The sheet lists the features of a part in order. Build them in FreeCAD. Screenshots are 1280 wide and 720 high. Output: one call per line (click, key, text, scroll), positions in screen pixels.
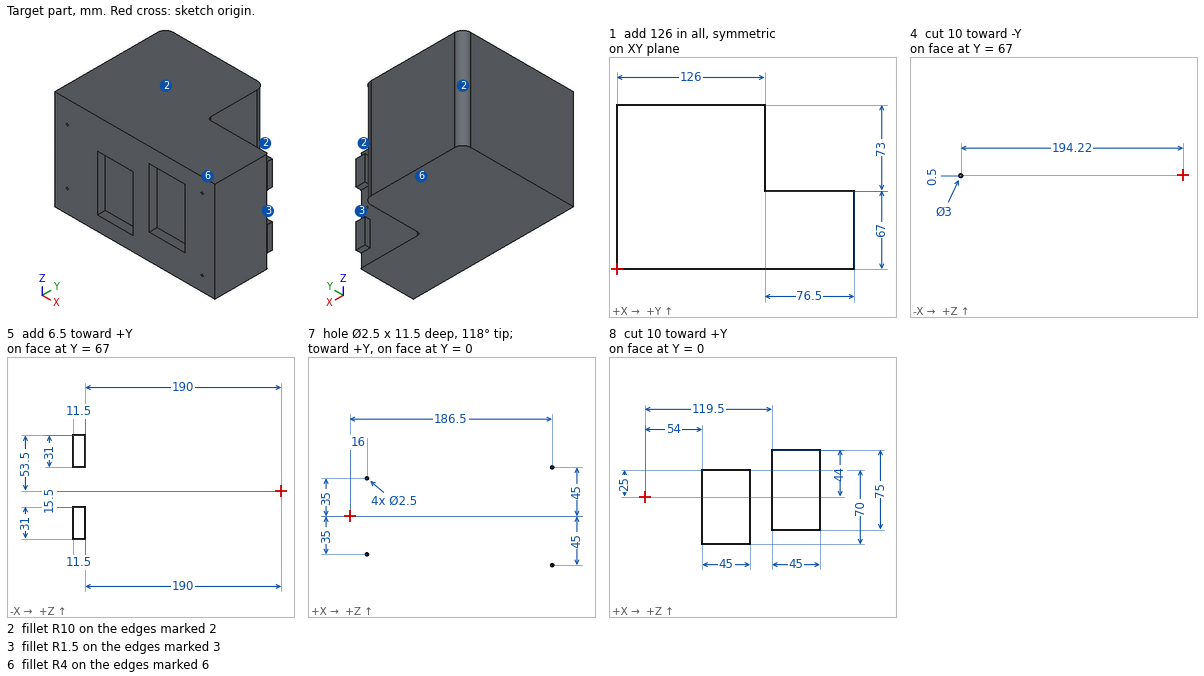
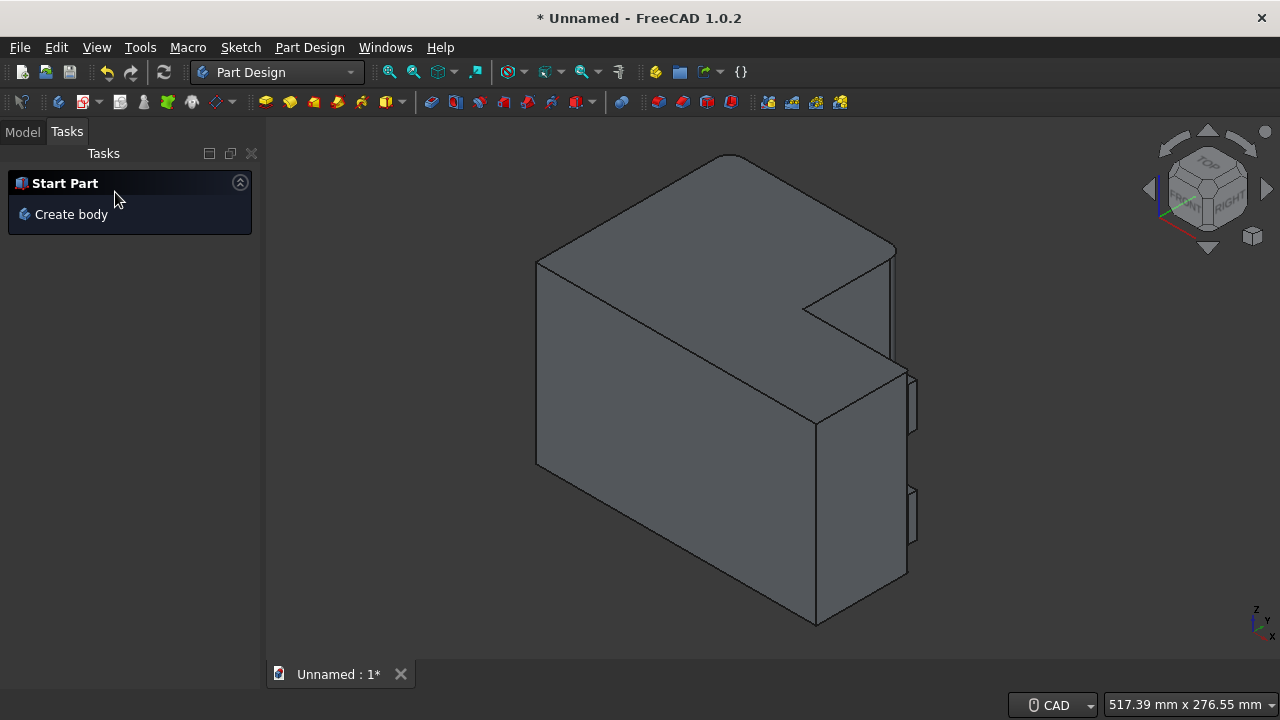
key(2)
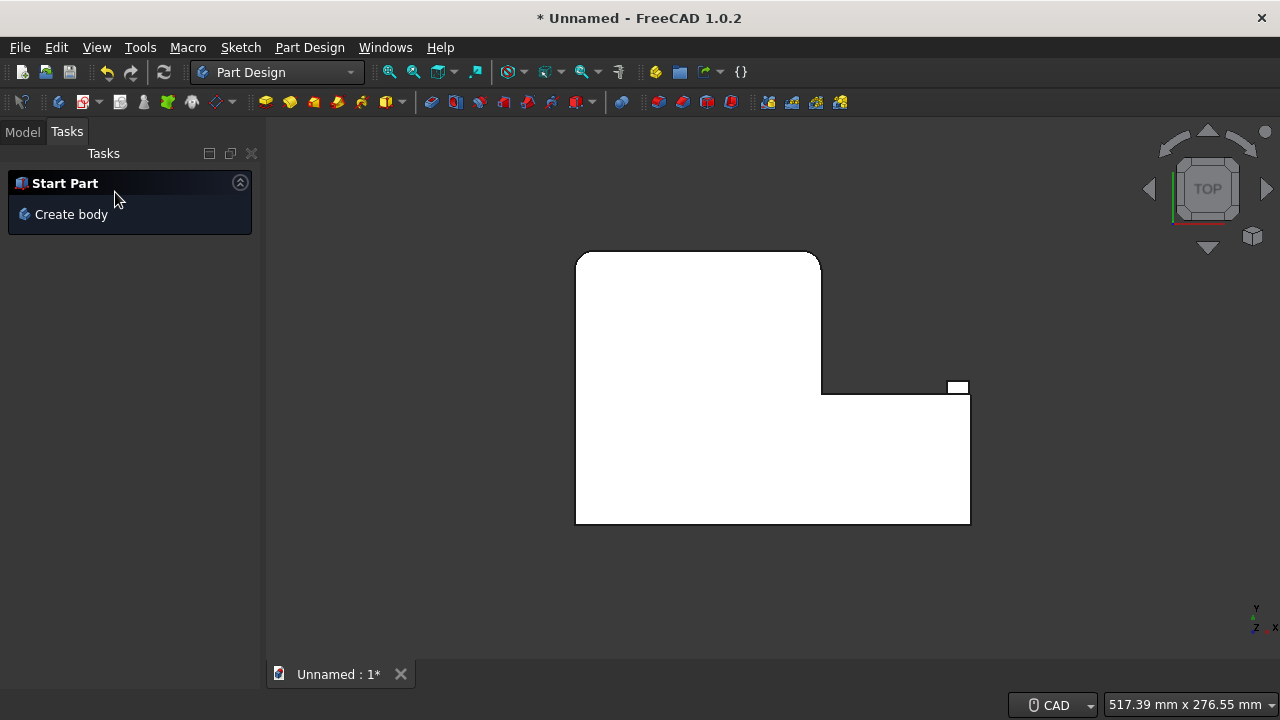
key(1)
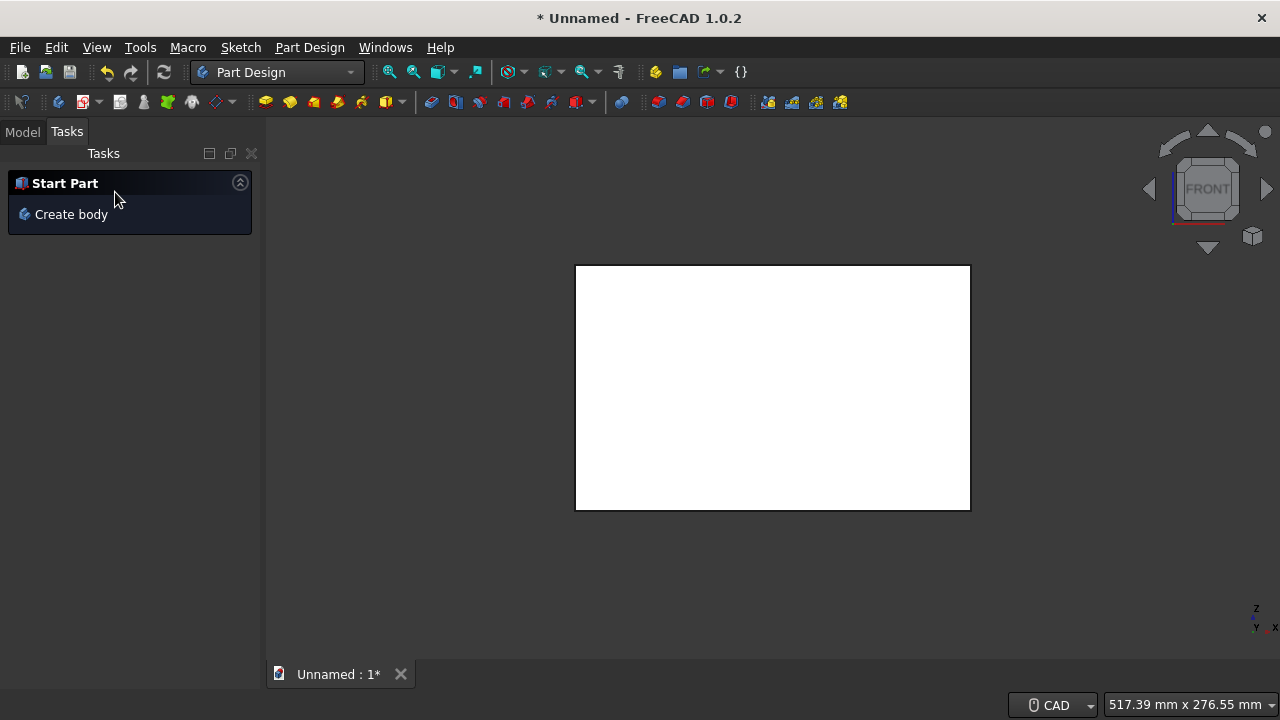
key(3)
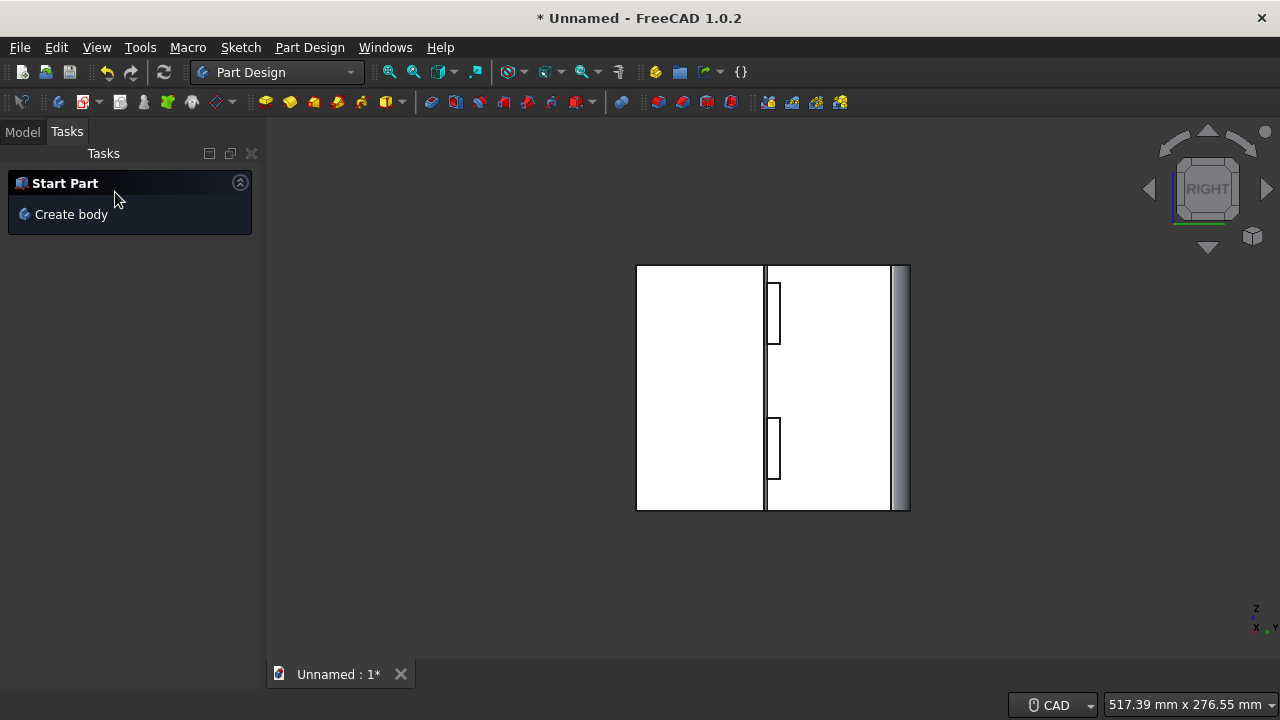
key(5)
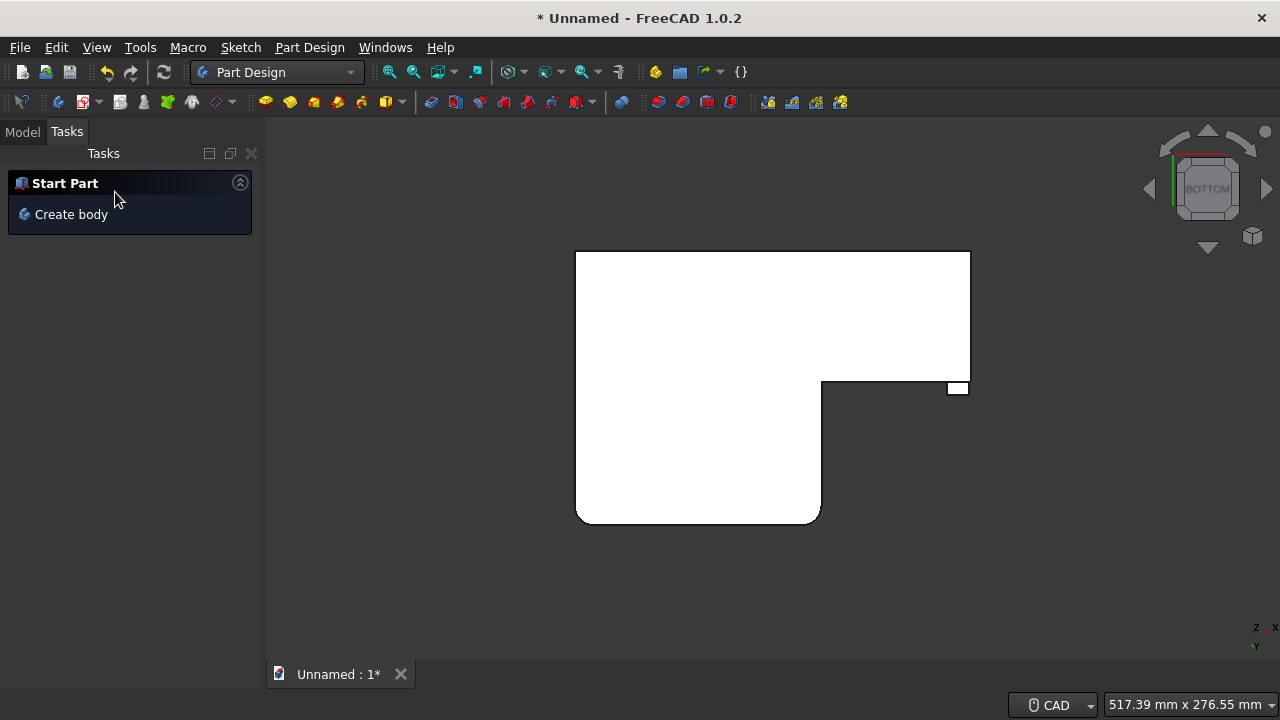
key(4)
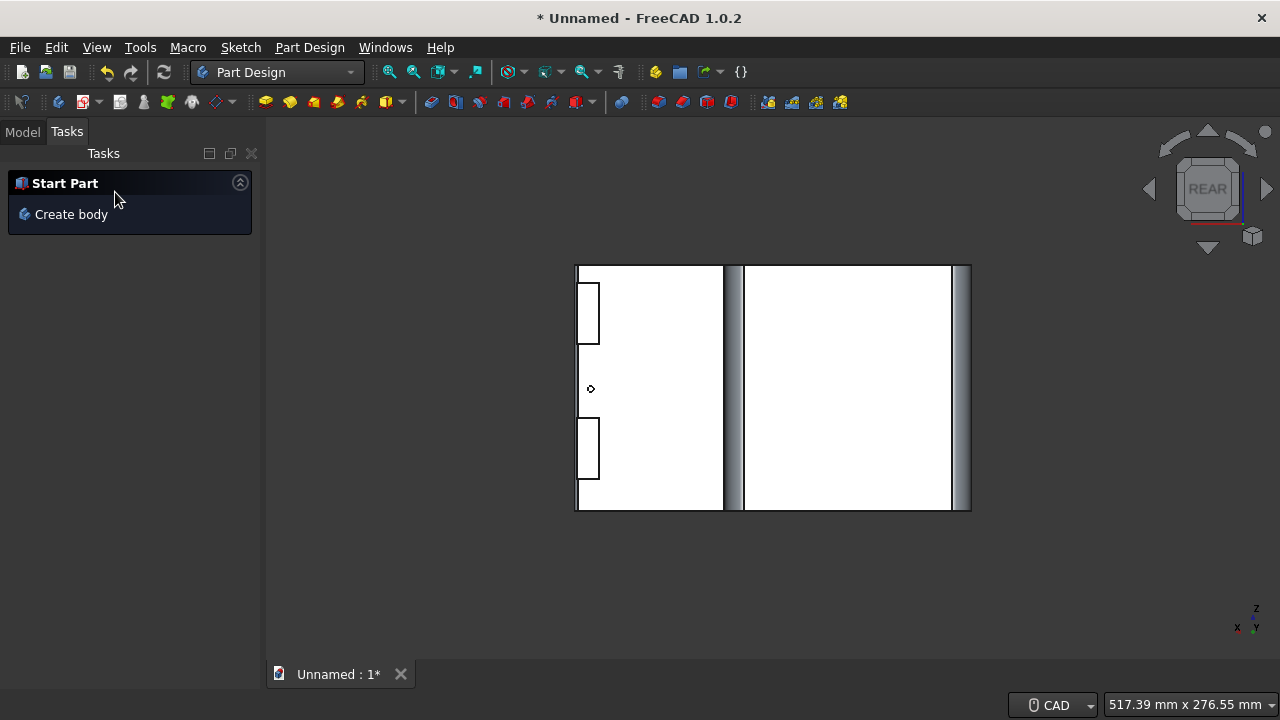
key(6)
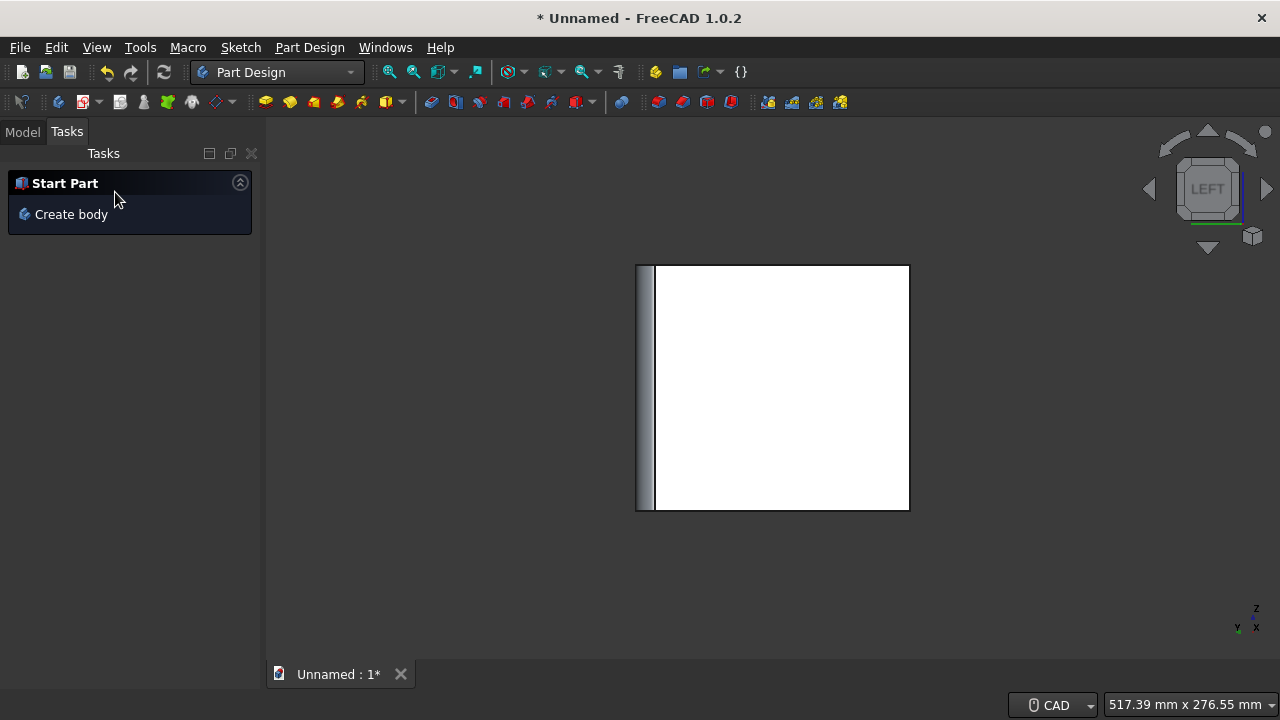
key(v)
key(3)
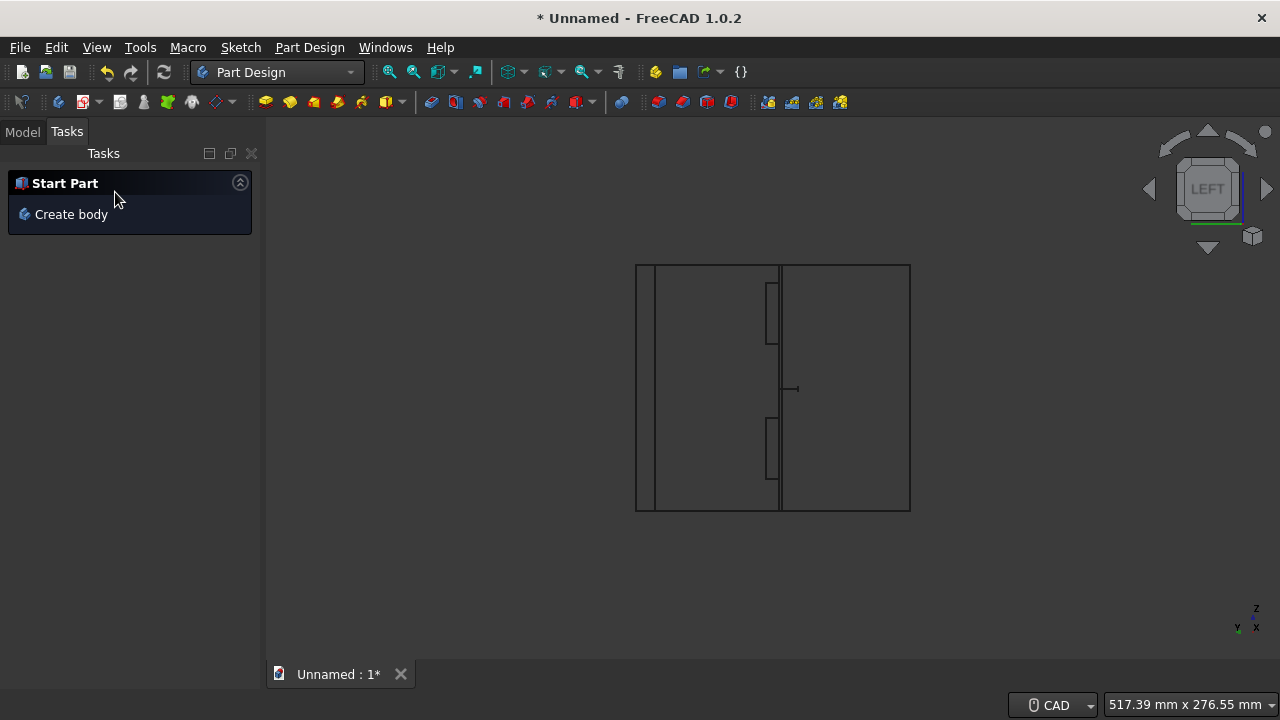
key(0)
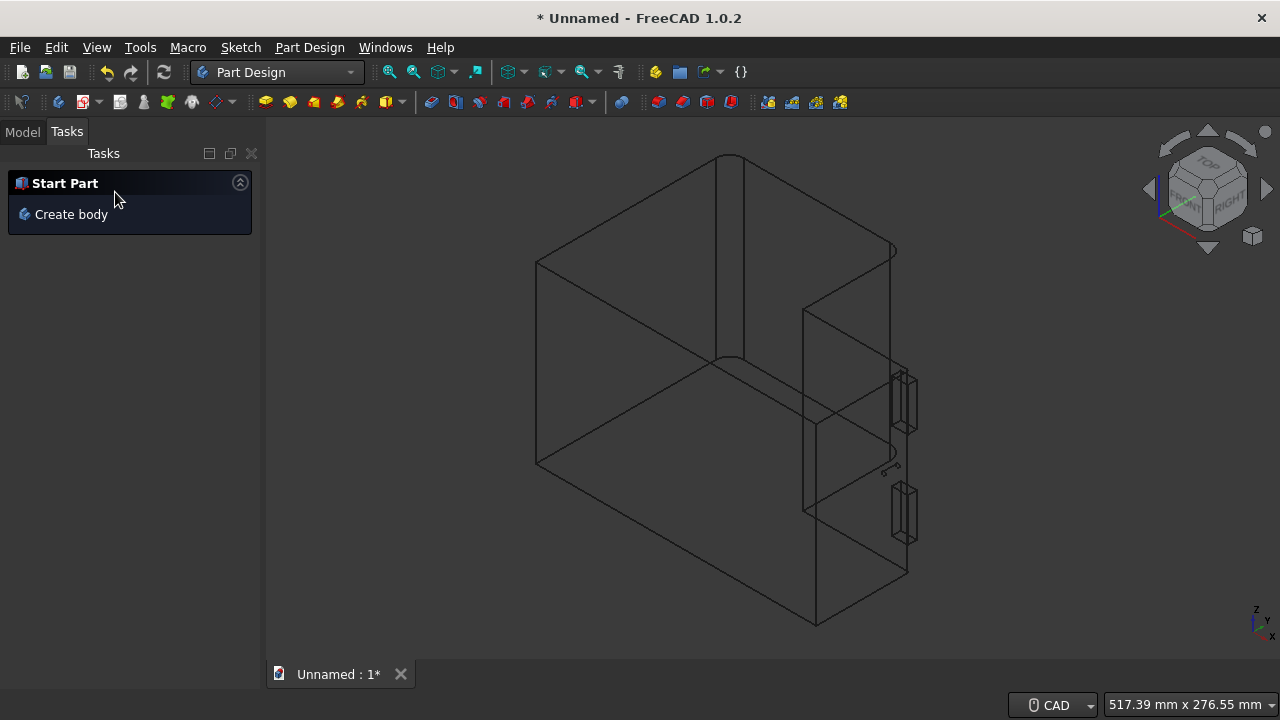
click(803, 429)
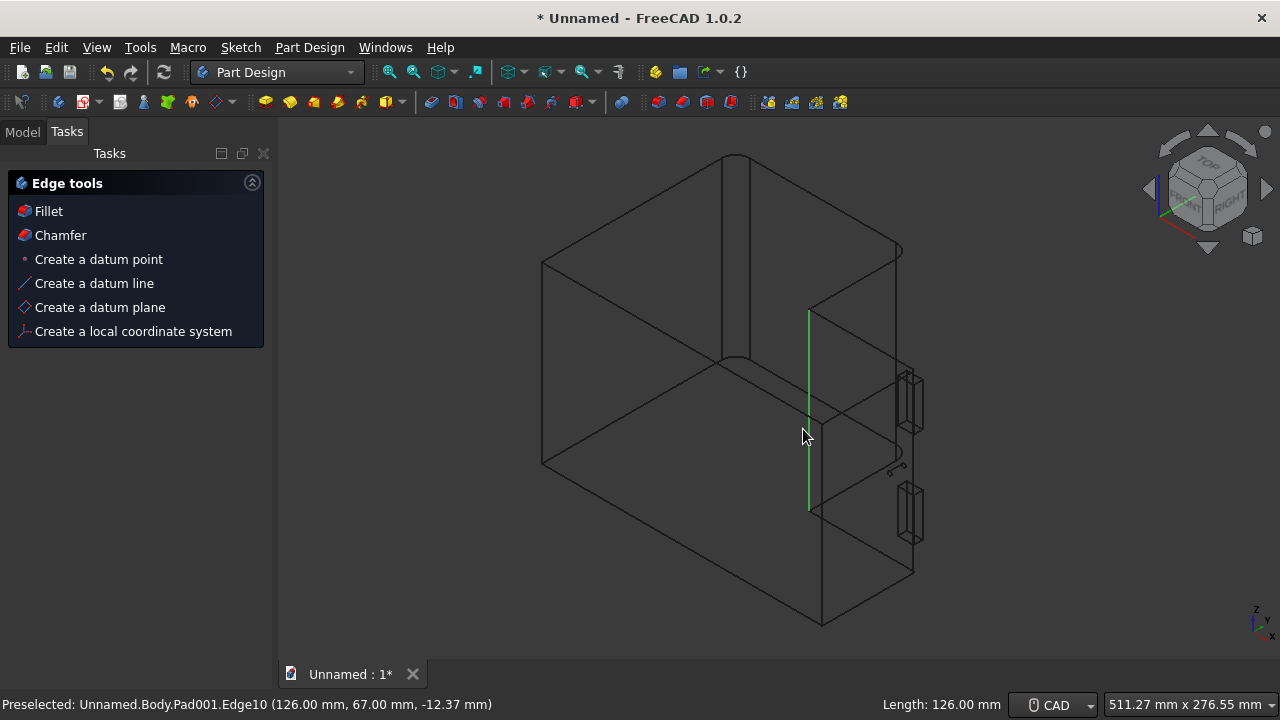
key(v)
key(1)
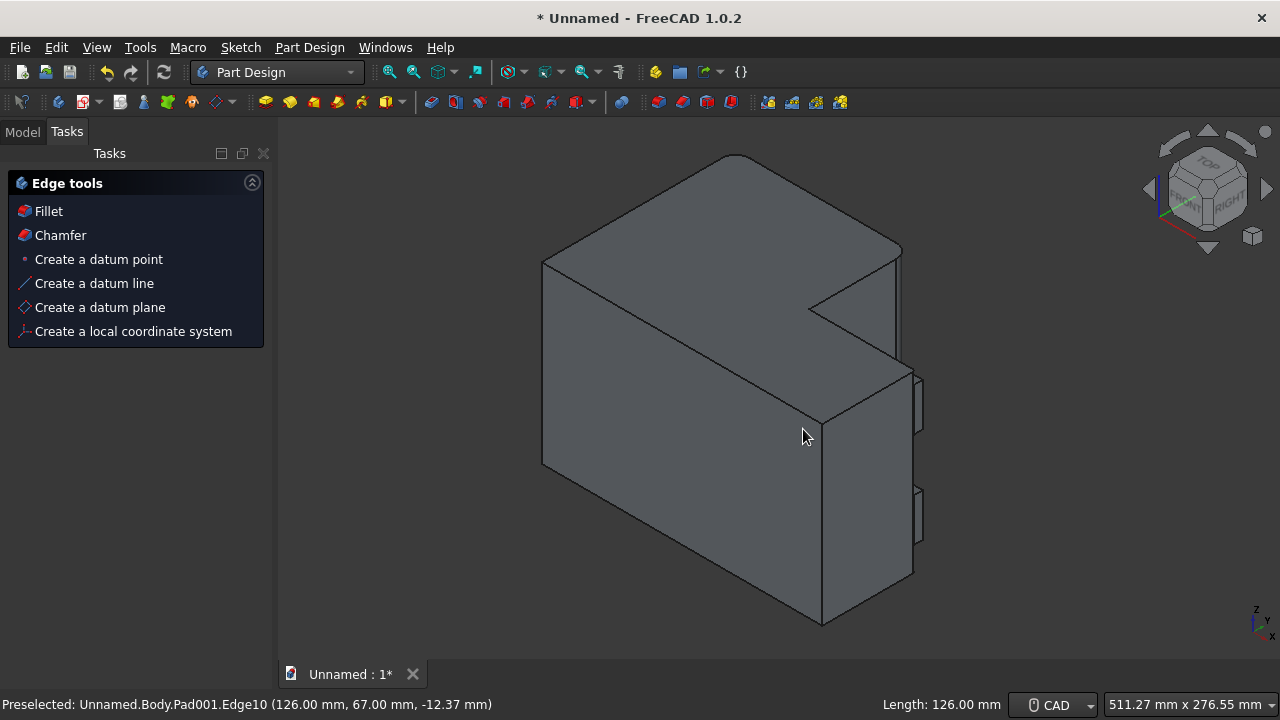
click(660, 102)